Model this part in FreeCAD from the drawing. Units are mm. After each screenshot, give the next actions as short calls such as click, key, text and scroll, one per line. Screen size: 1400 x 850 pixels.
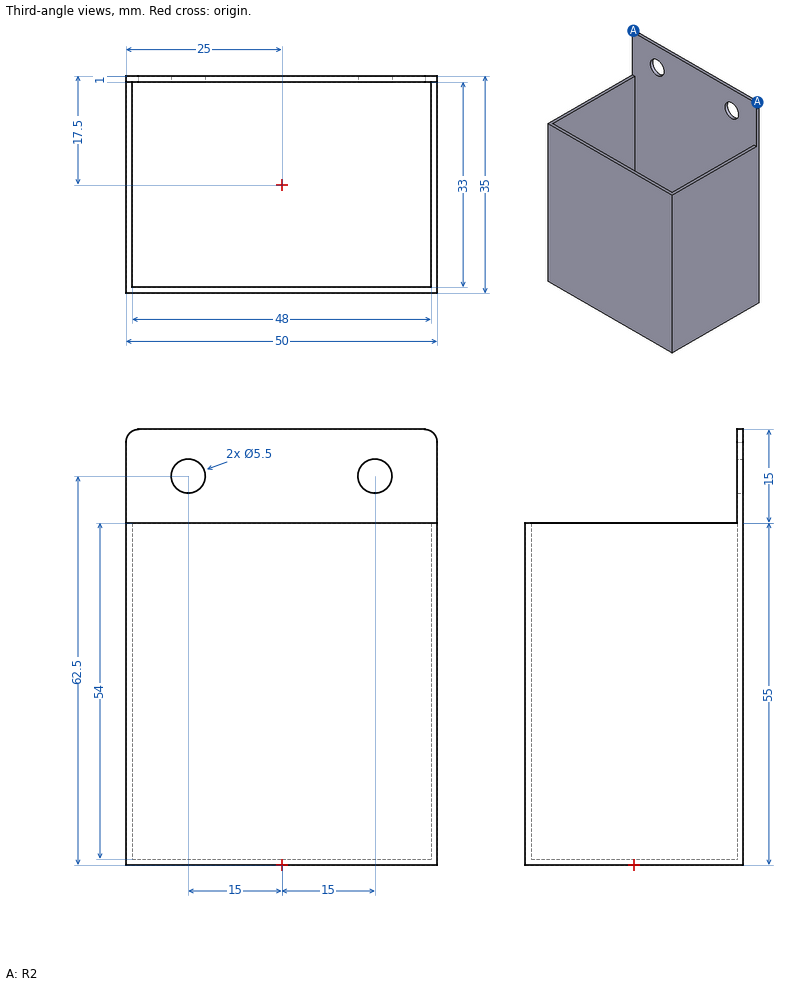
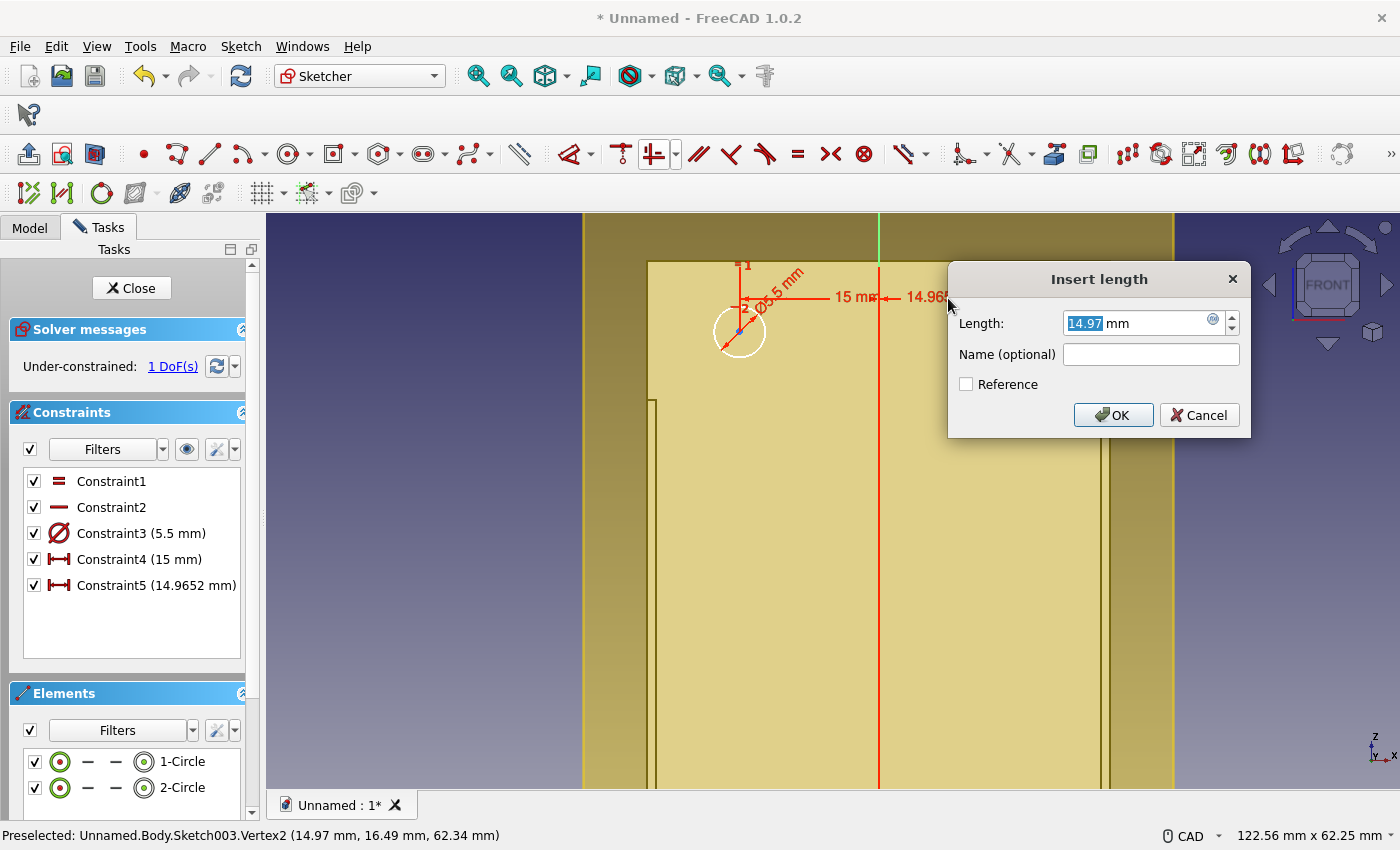
text(15)
key(Return)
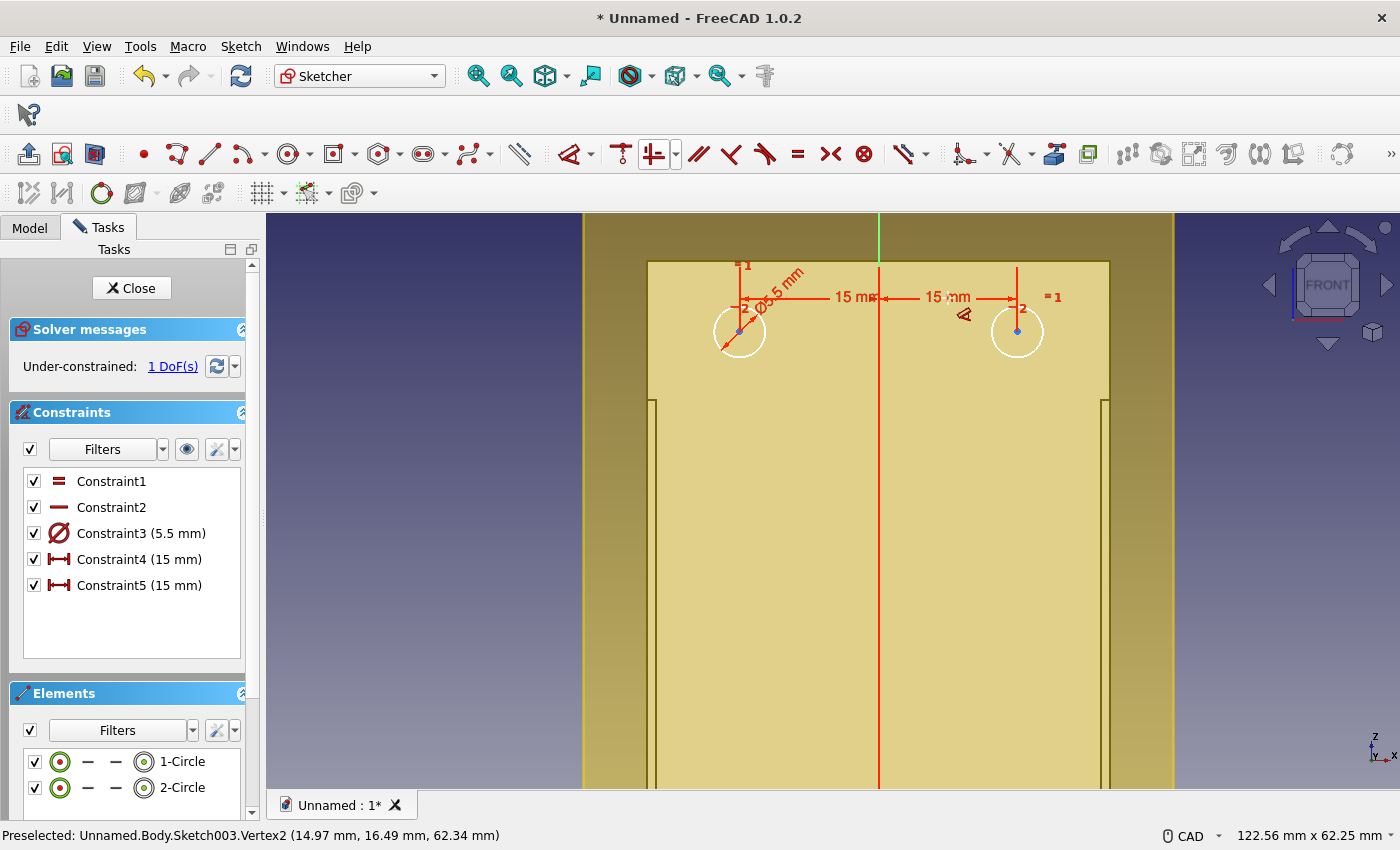
click(740, 332)
click(706, 547)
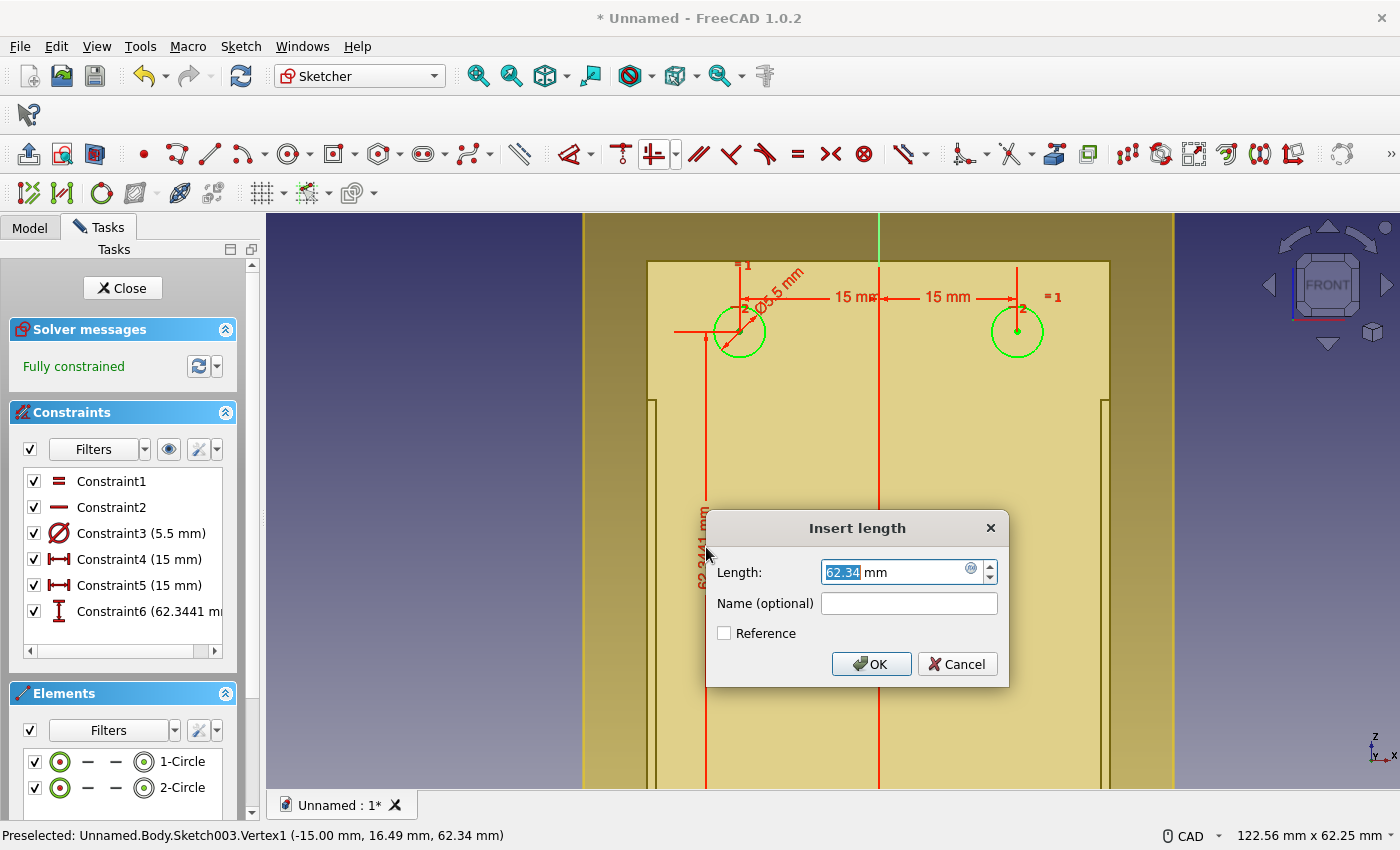
text(62.5)
key(Return)
key(Escape)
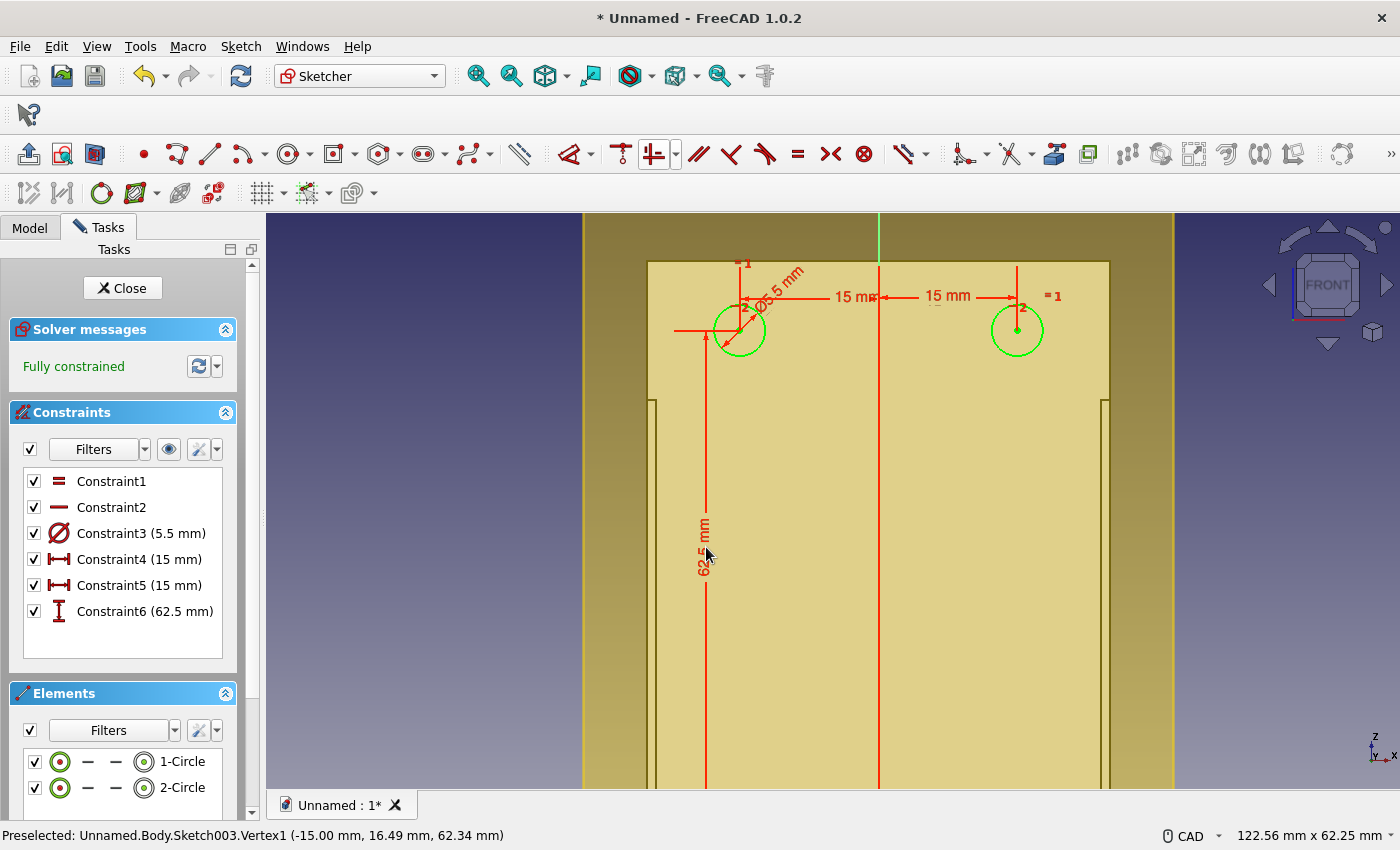
click(123, 288)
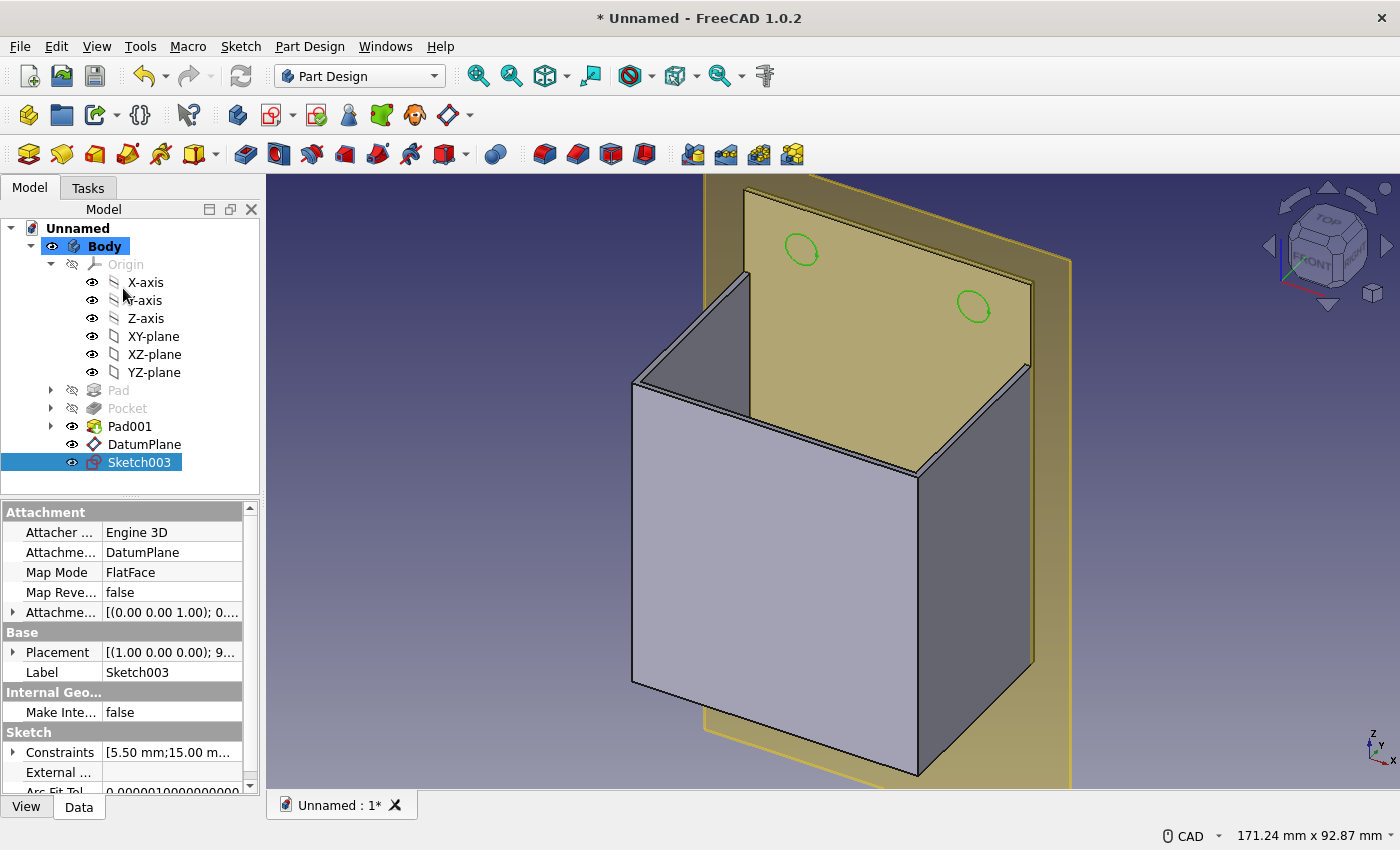
click(246, 154)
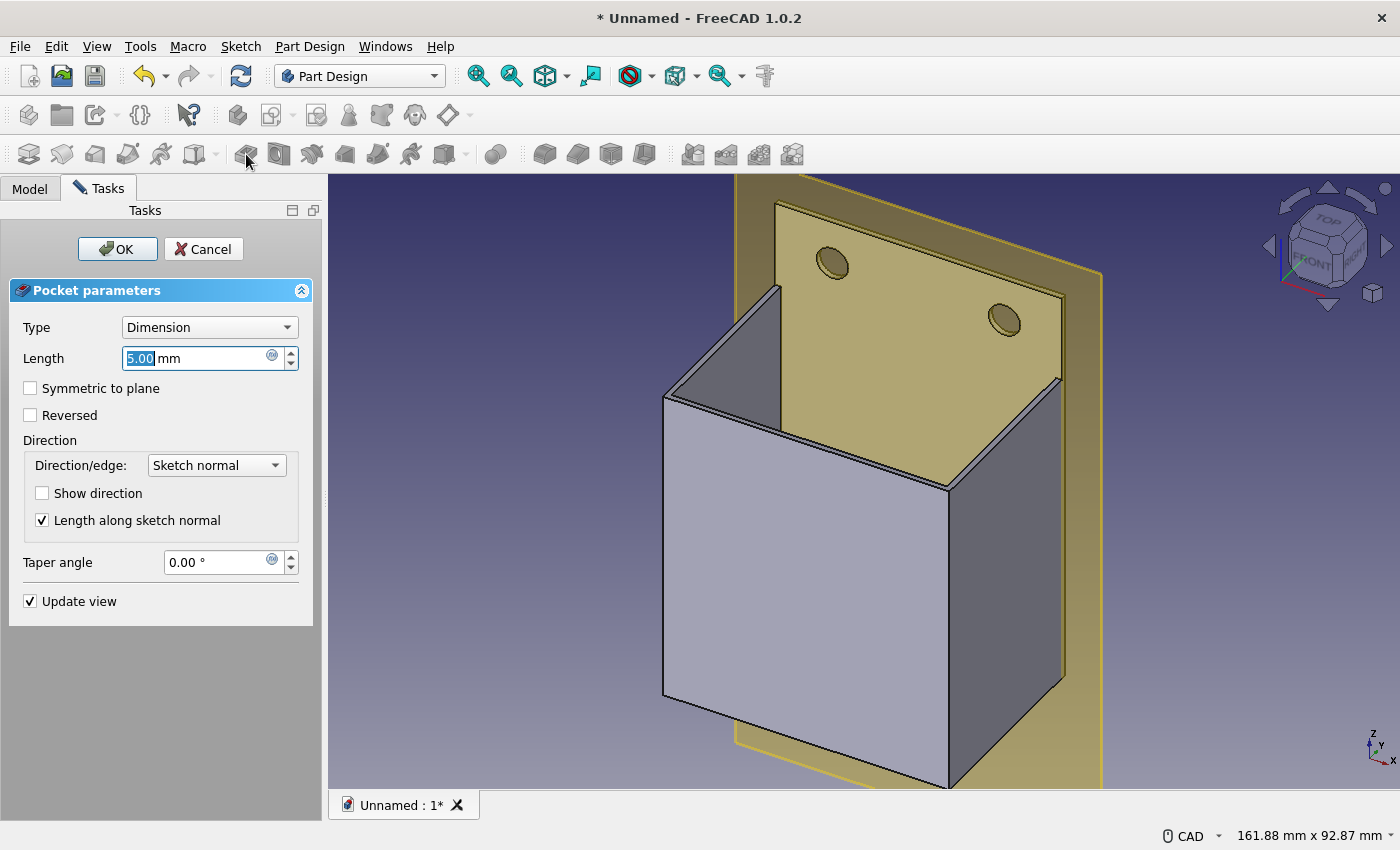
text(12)
key(Tab)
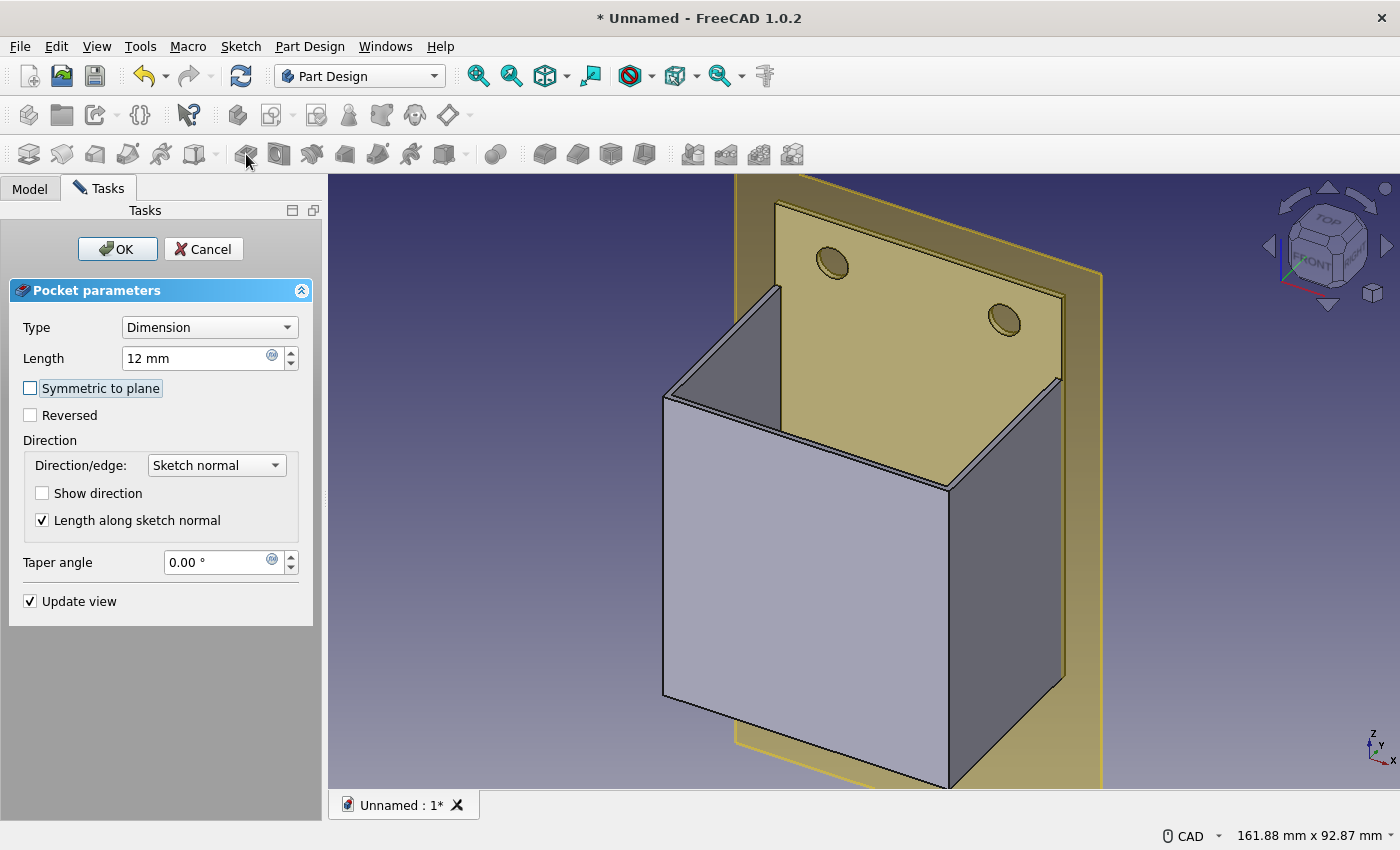
click(118, 249)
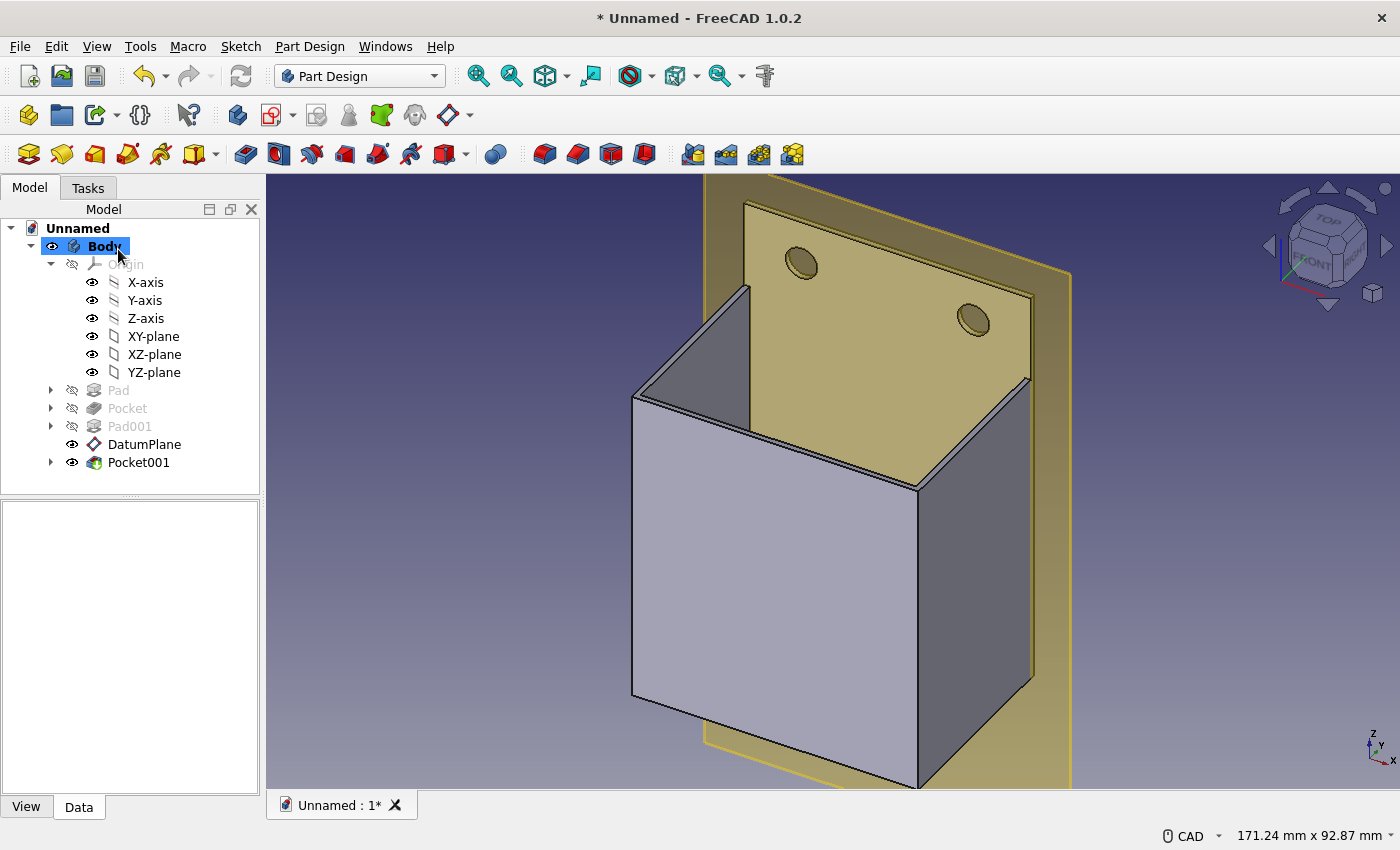
click(117, 444)
key(space)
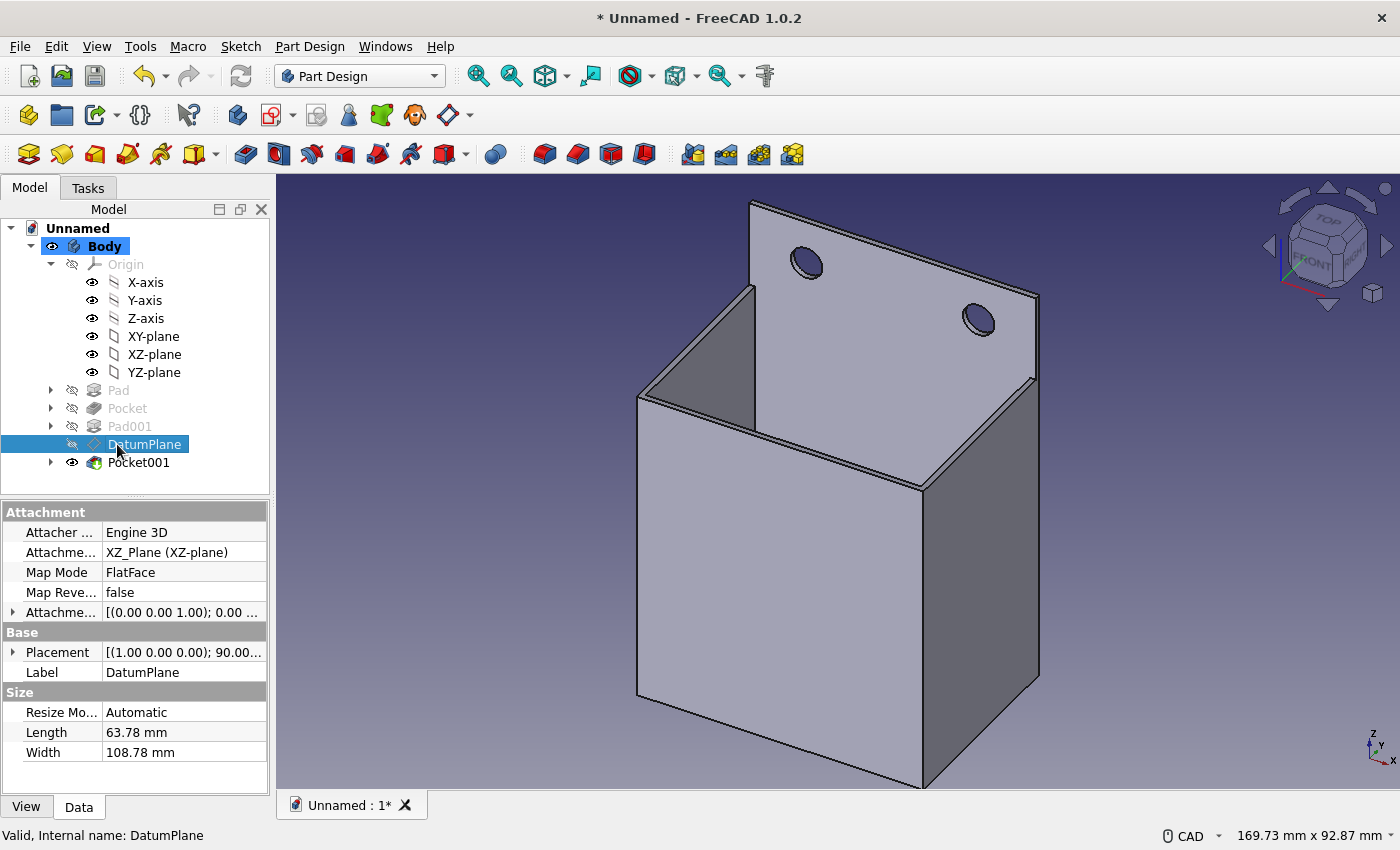
scroll(1038, 296, up, 9)